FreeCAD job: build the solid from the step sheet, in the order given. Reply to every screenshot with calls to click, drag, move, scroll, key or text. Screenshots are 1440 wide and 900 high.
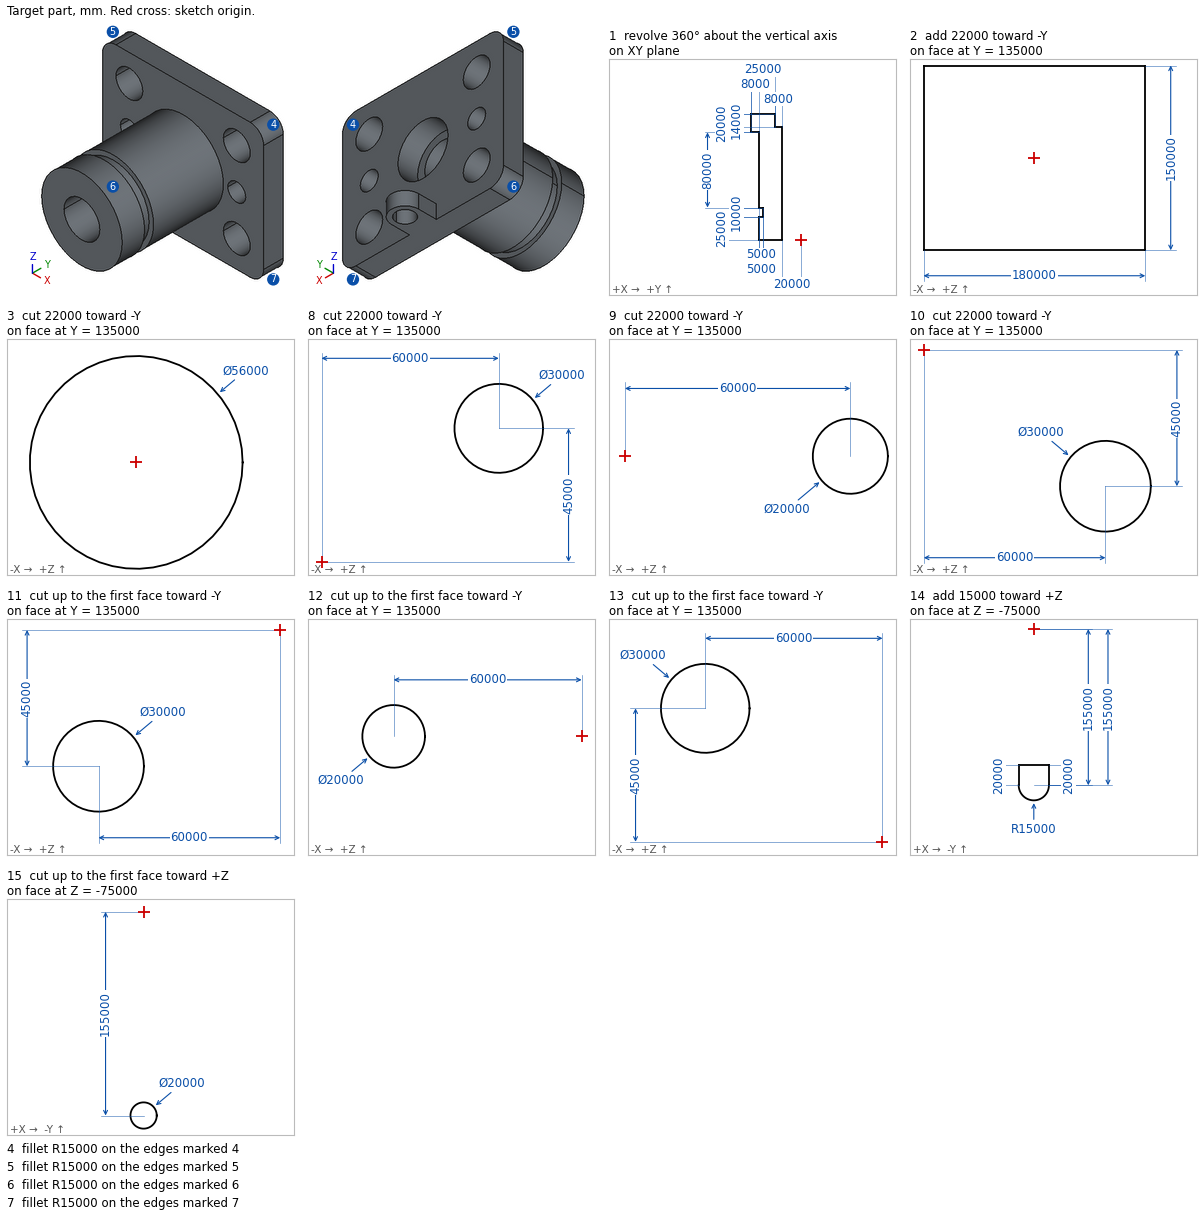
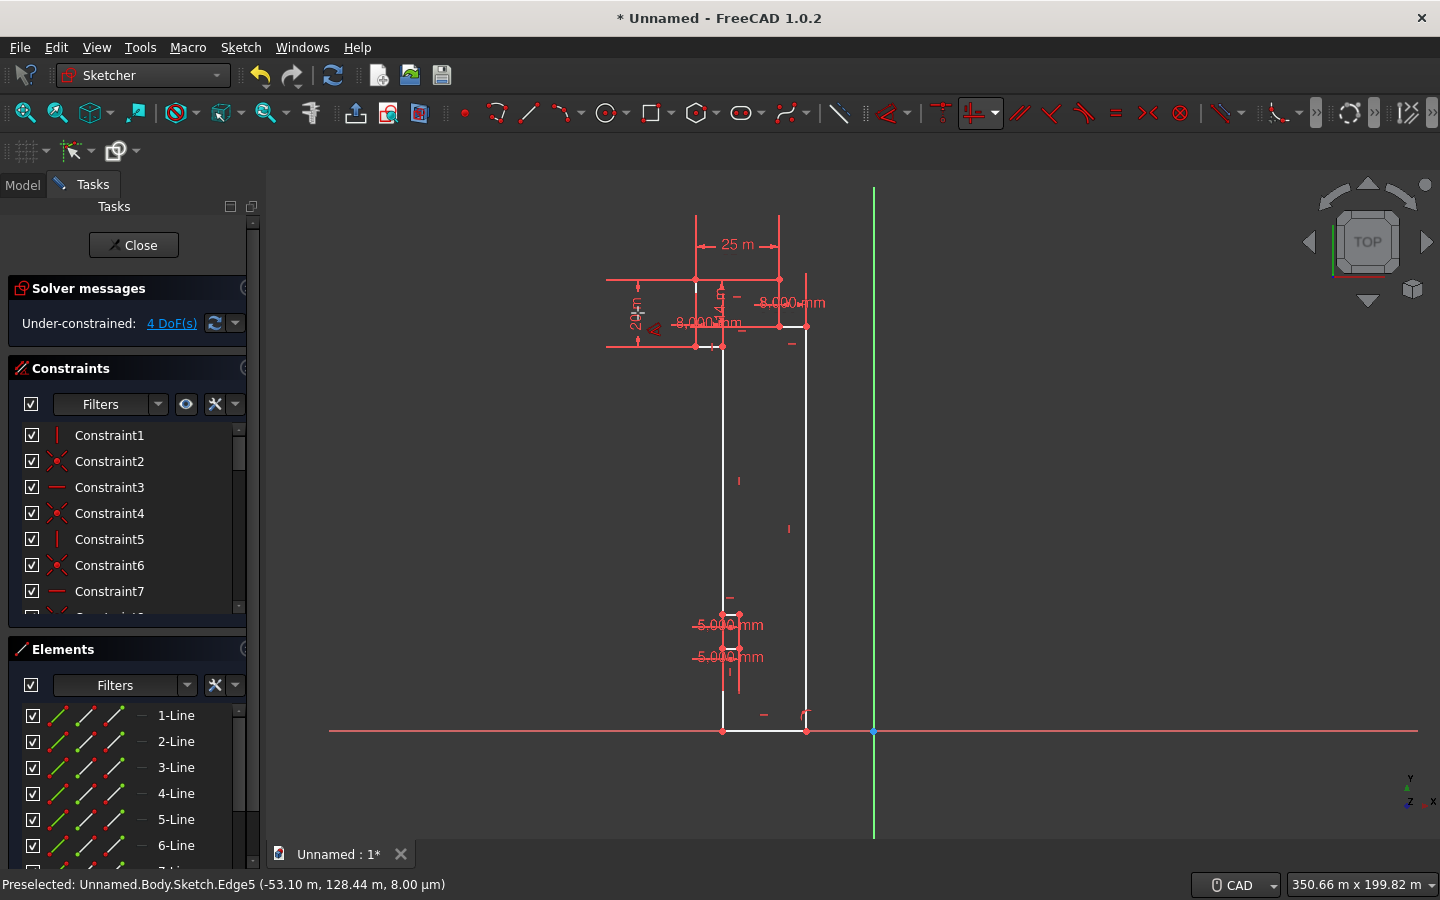
click(723, 427)
click(689, 481)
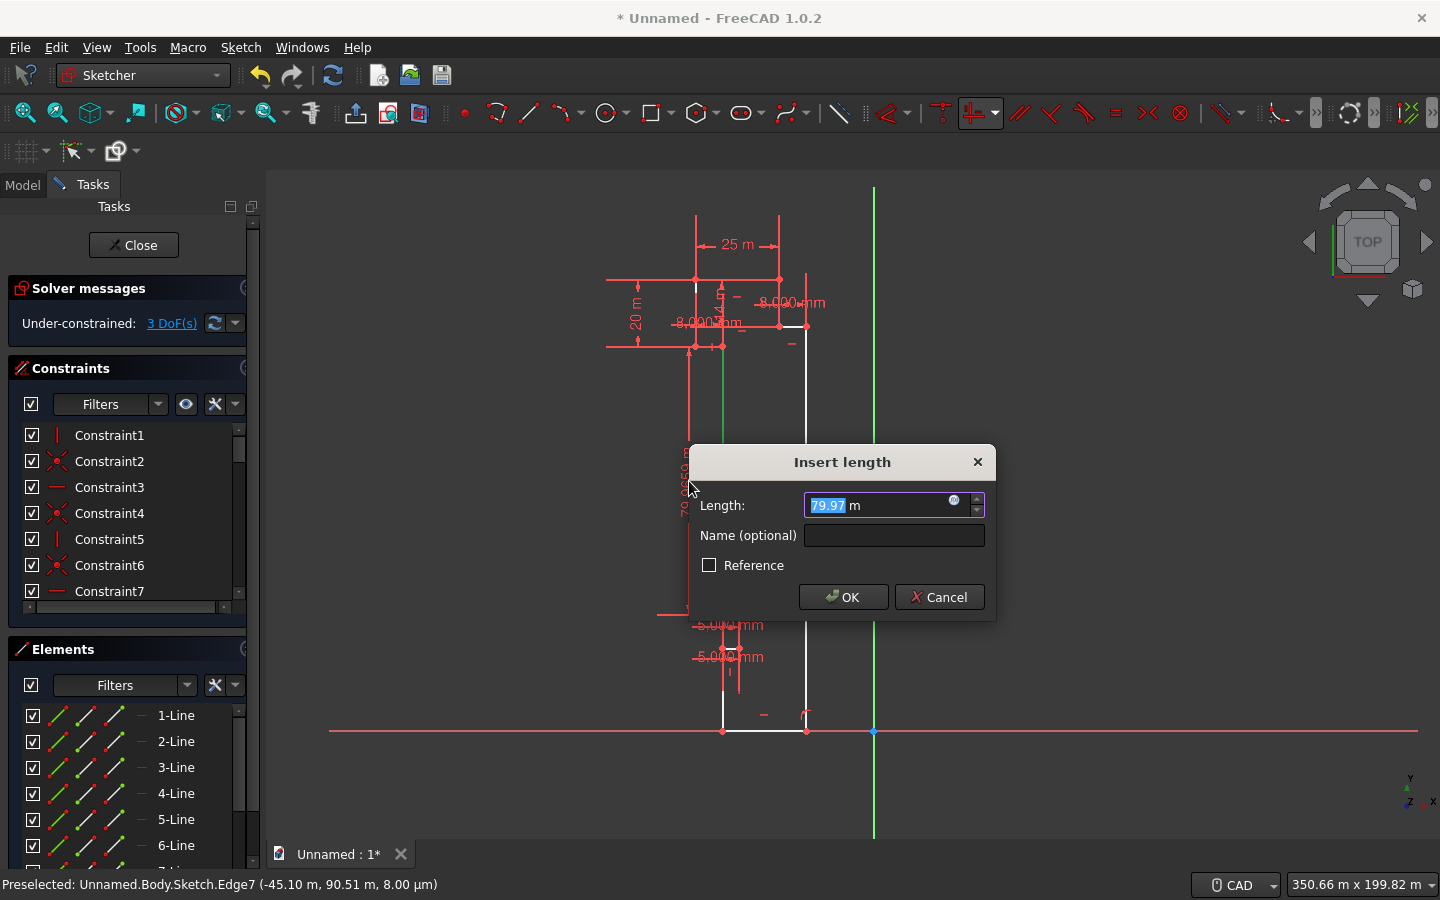
key(ctrl+a)
text(80000 mm)
key(Return)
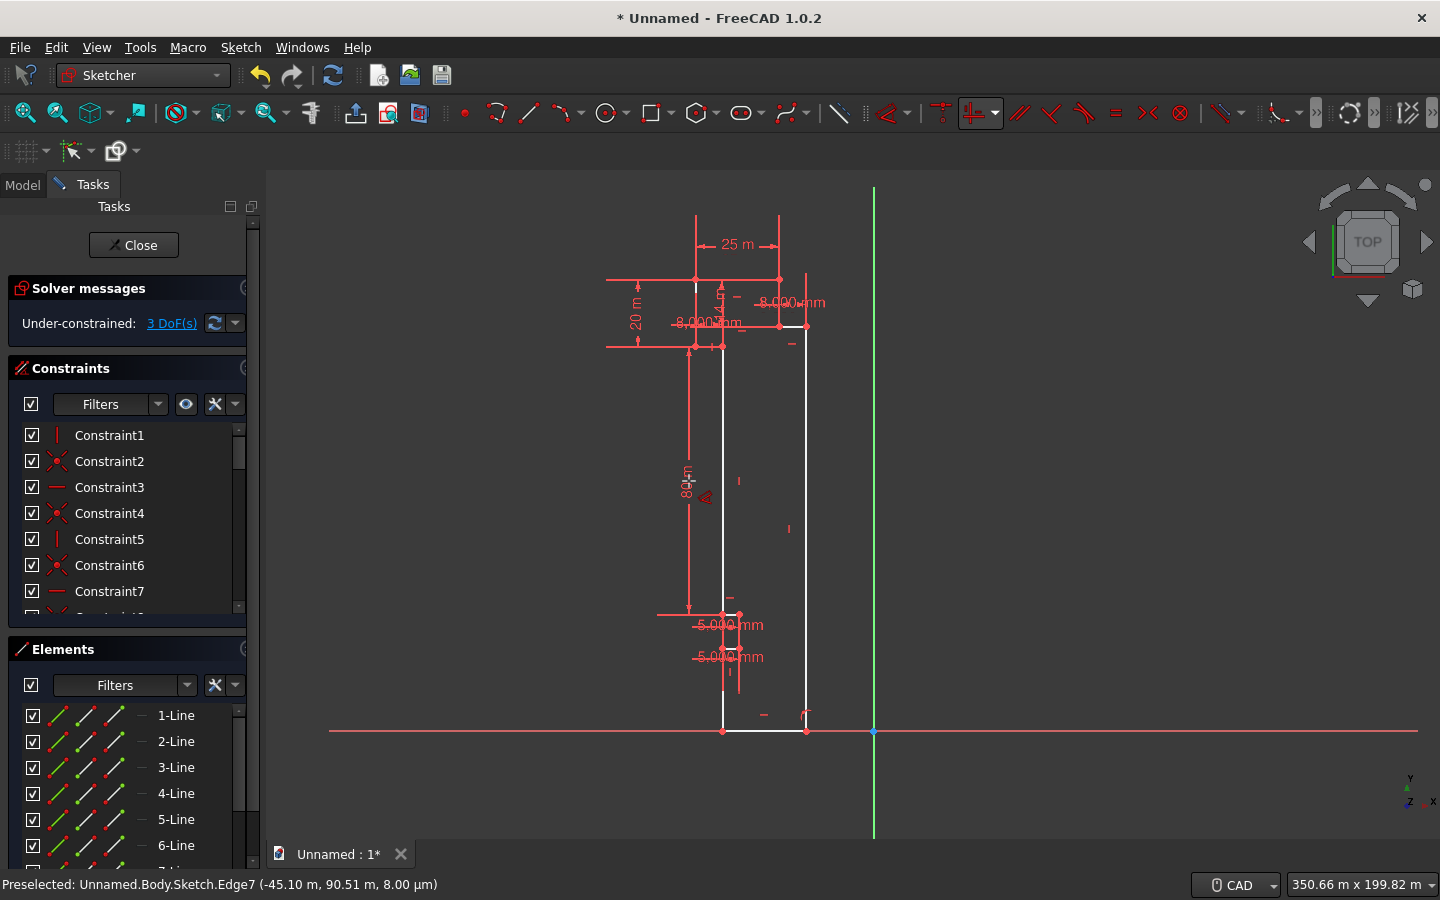
scroll(739, 625, up, 2)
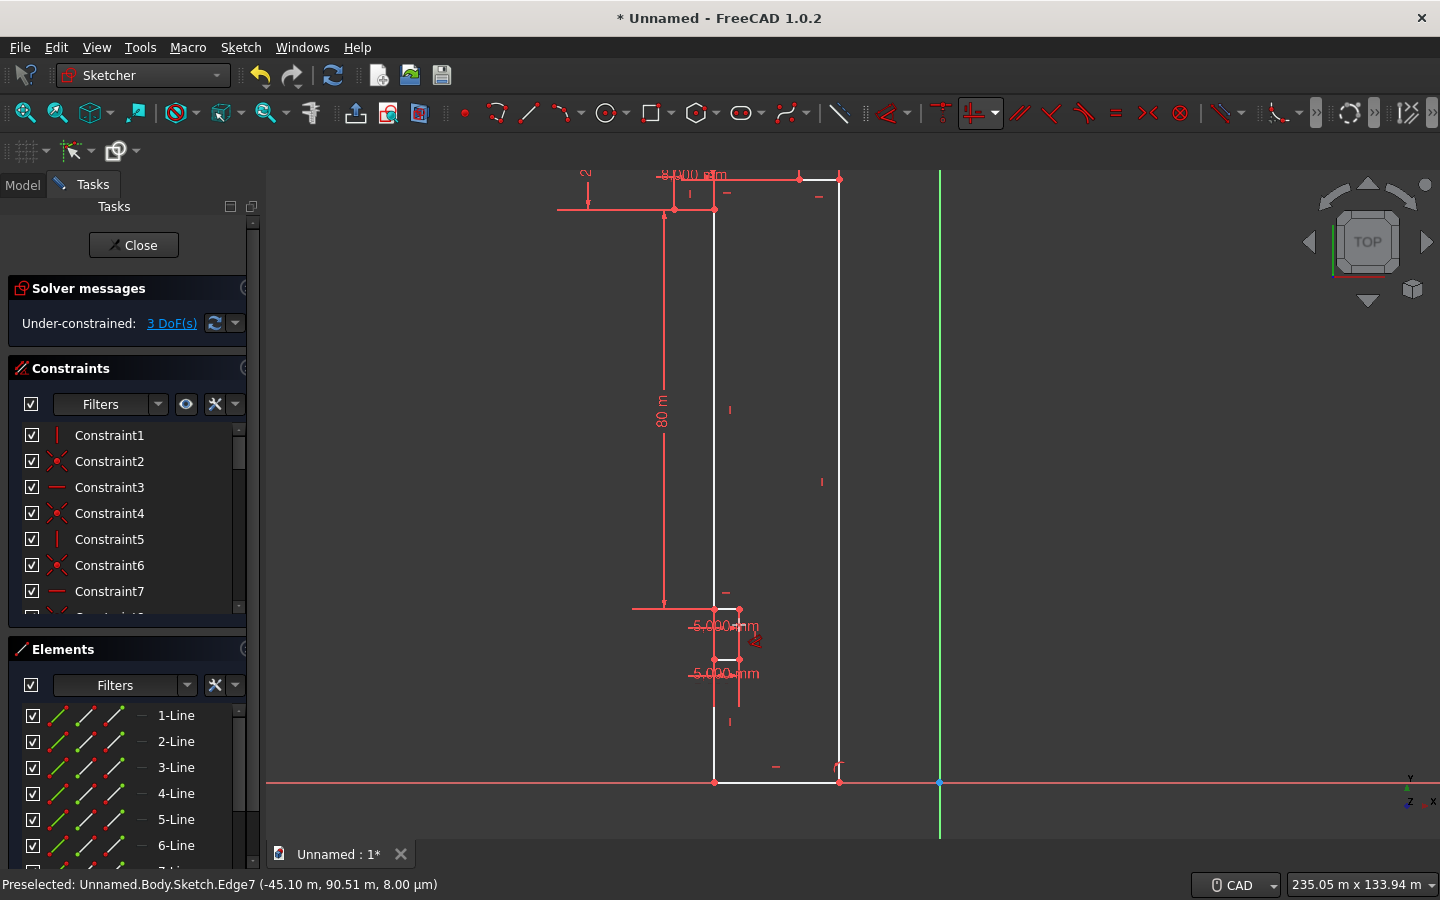
click(739, 624)
click(773, 652)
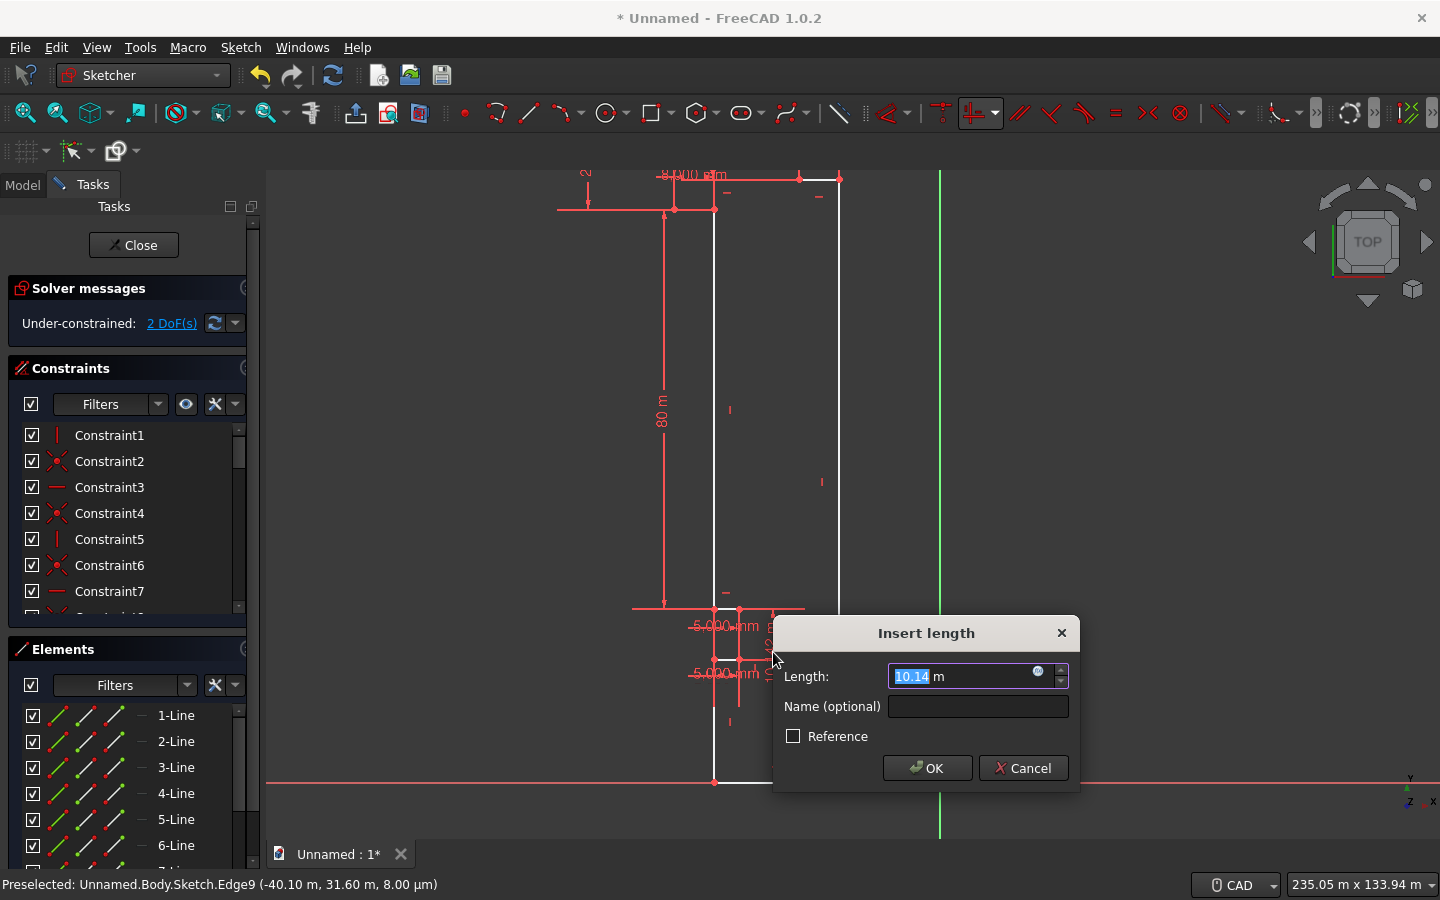
key(ctrl+a)
text(10000 mm)
key(Return)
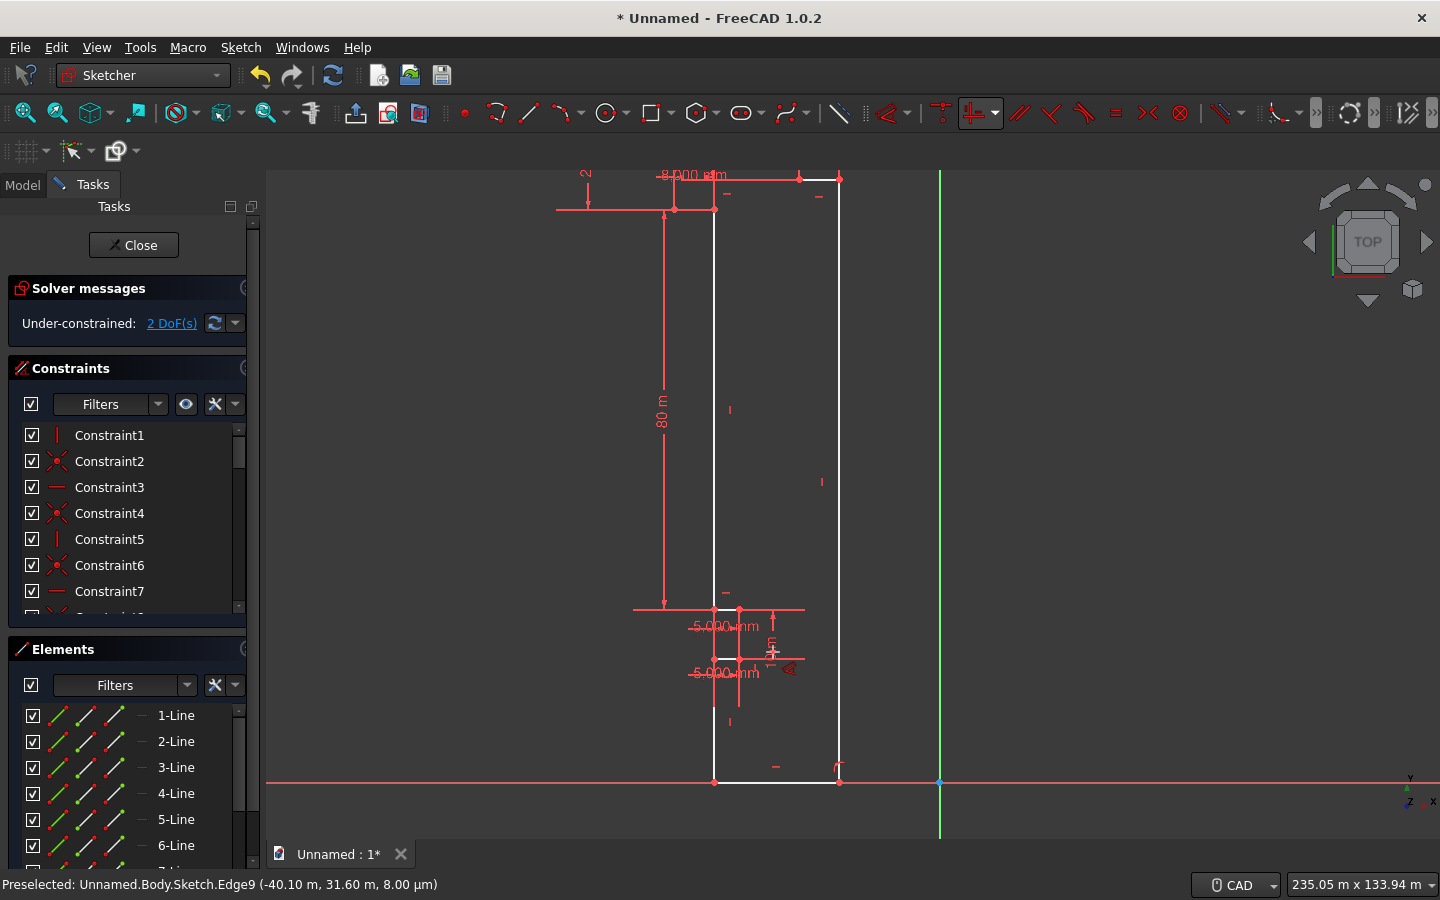
click(714, 696)
click(680, 721)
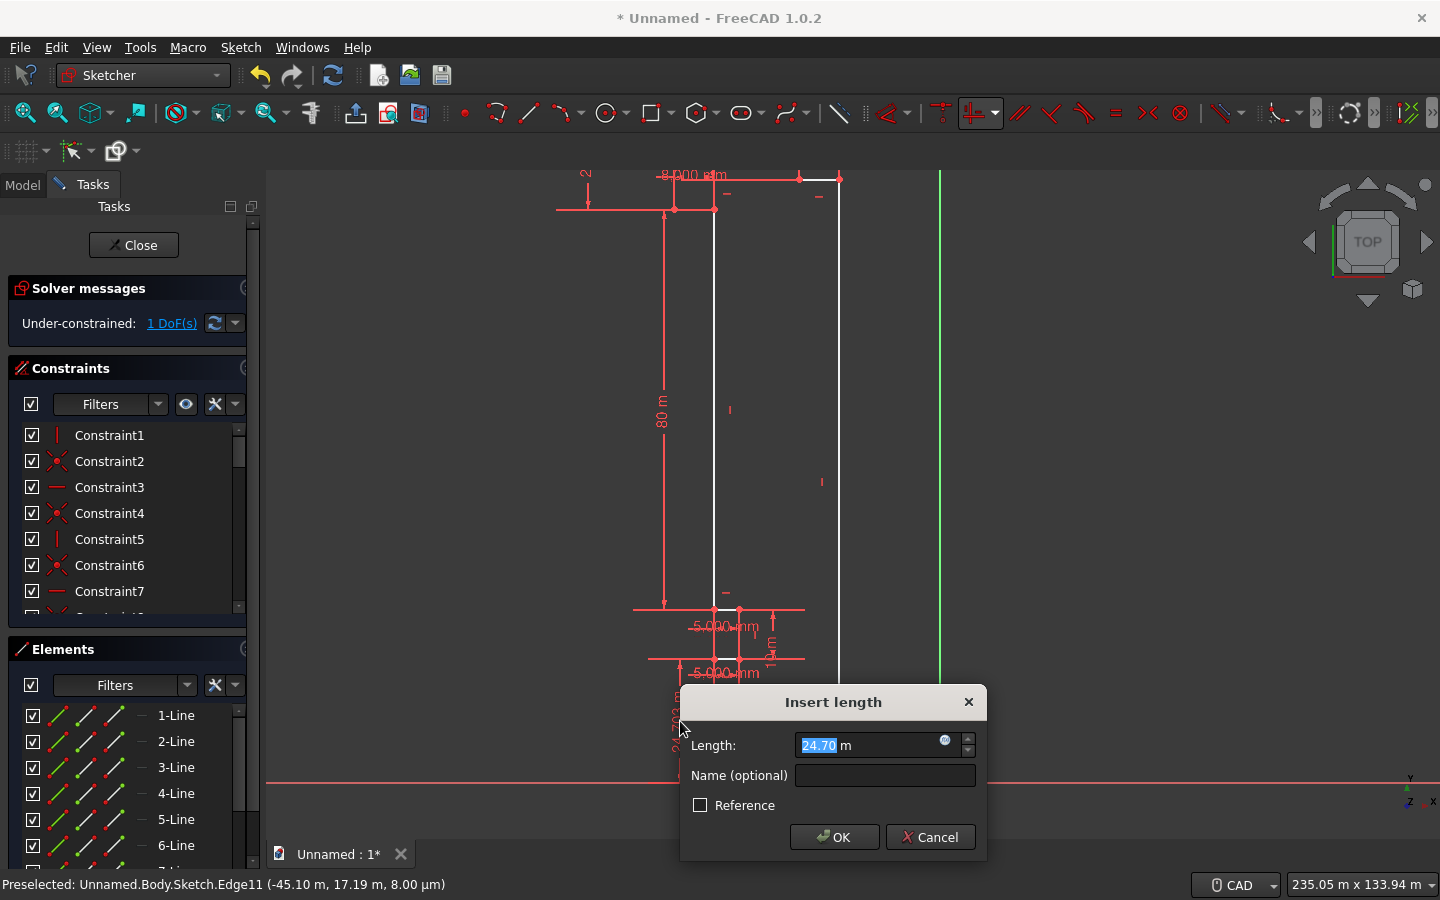
key(ctrl+a)
text(25000 mm)
key(Return)